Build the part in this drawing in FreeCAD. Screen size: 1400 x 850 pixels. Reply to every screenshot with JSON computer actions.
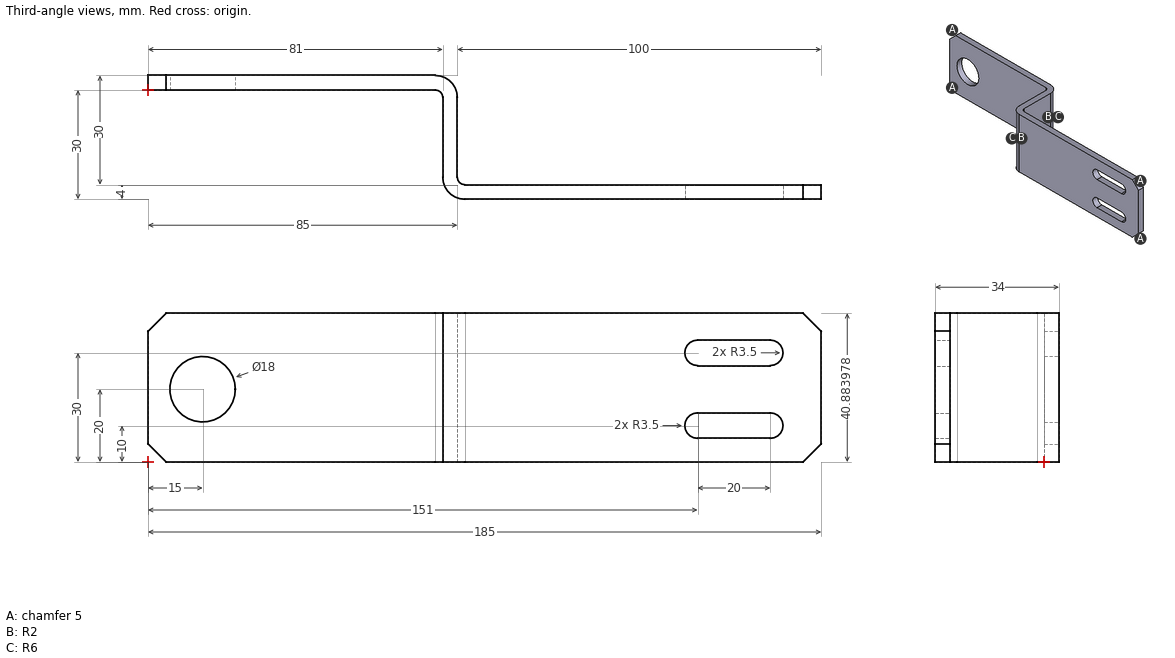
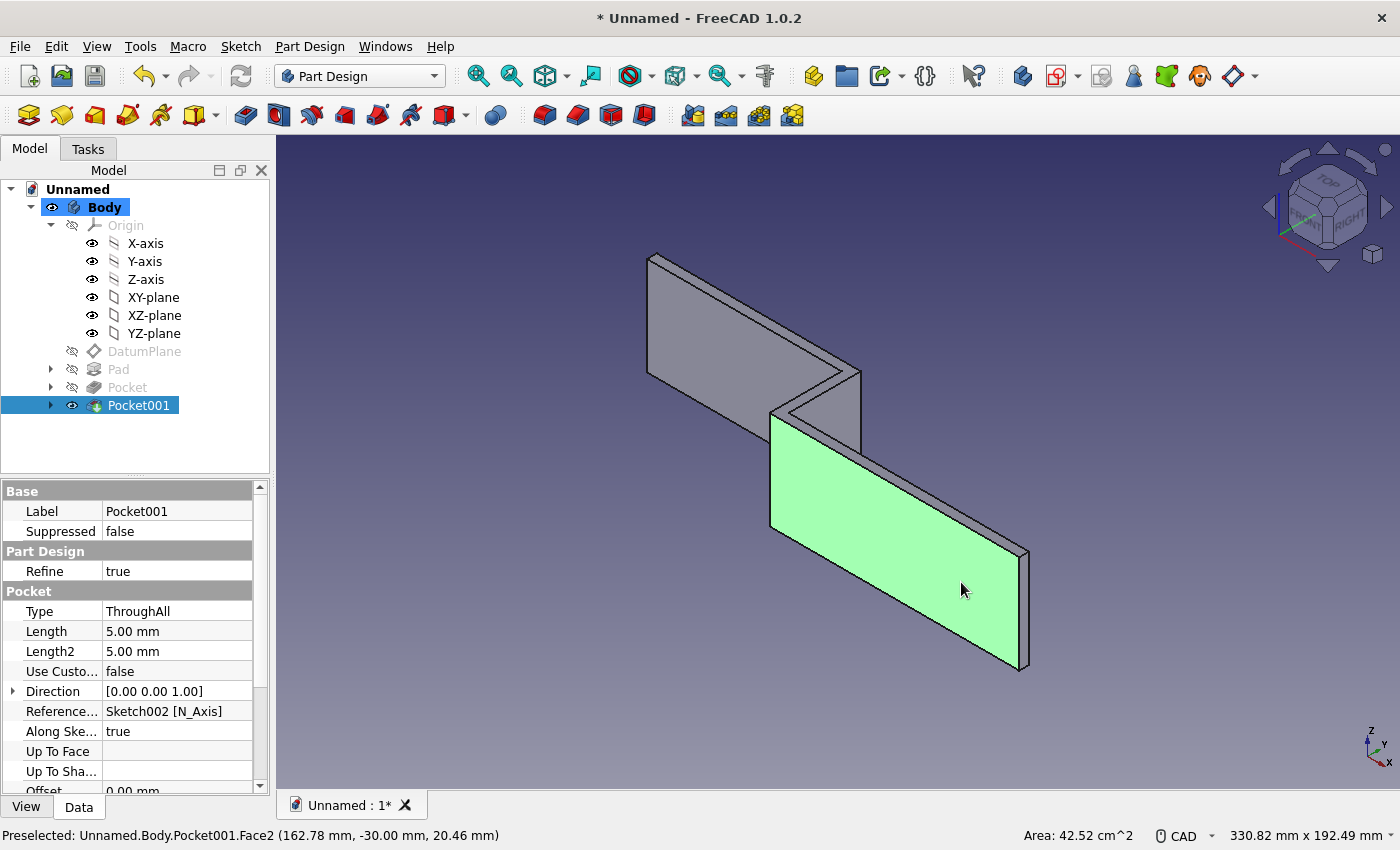
{"action": "left_click", "coordinate": [1056, 76]}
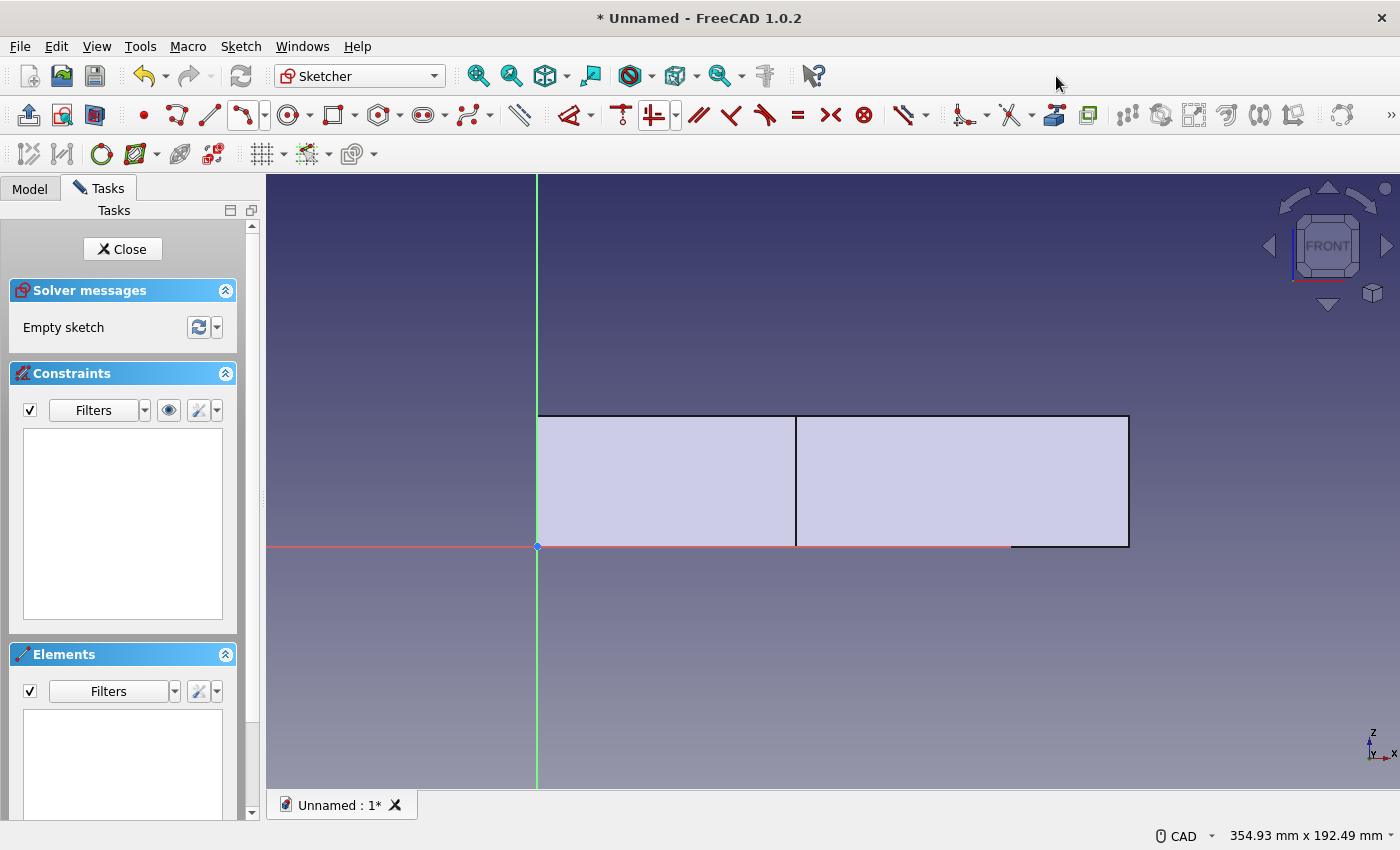
{"action": "scroll", "coordinate": [1097, 520], "scroll_direction": "up", "scroll_amount": 10}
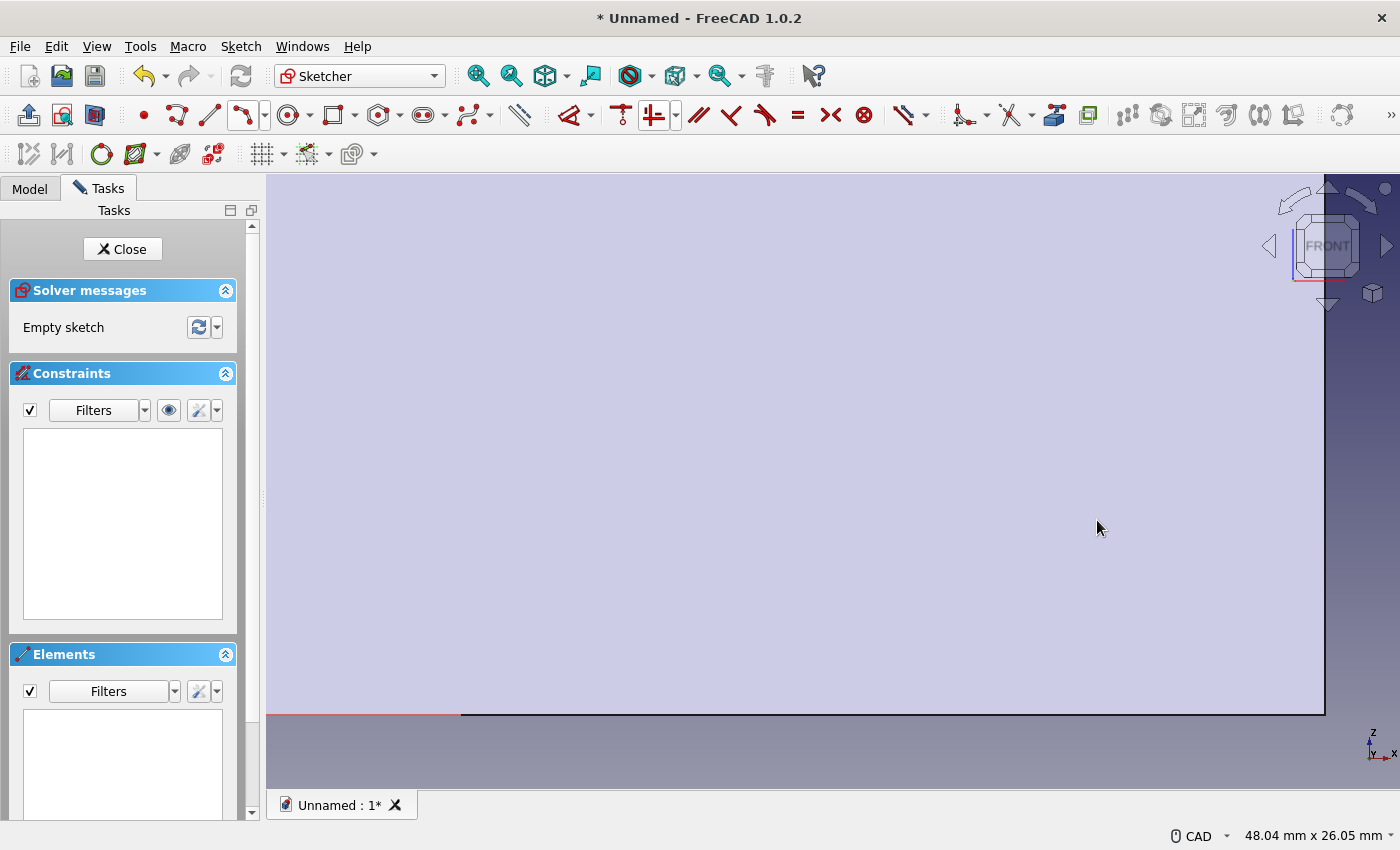
{"action": "left_click", "coordinate": [422, 116]}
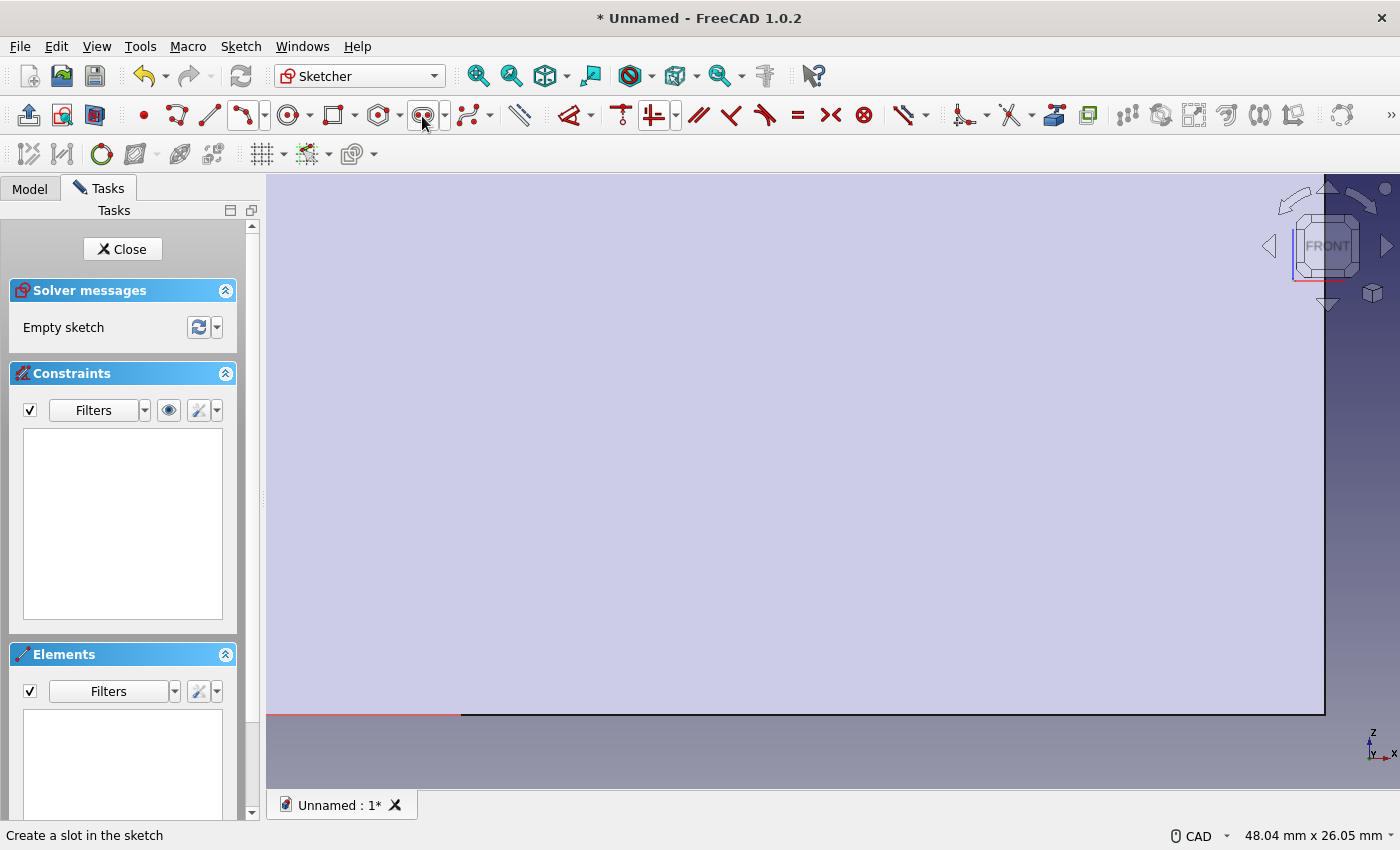
{"action": "left_click", "coordinate": [523, 478]}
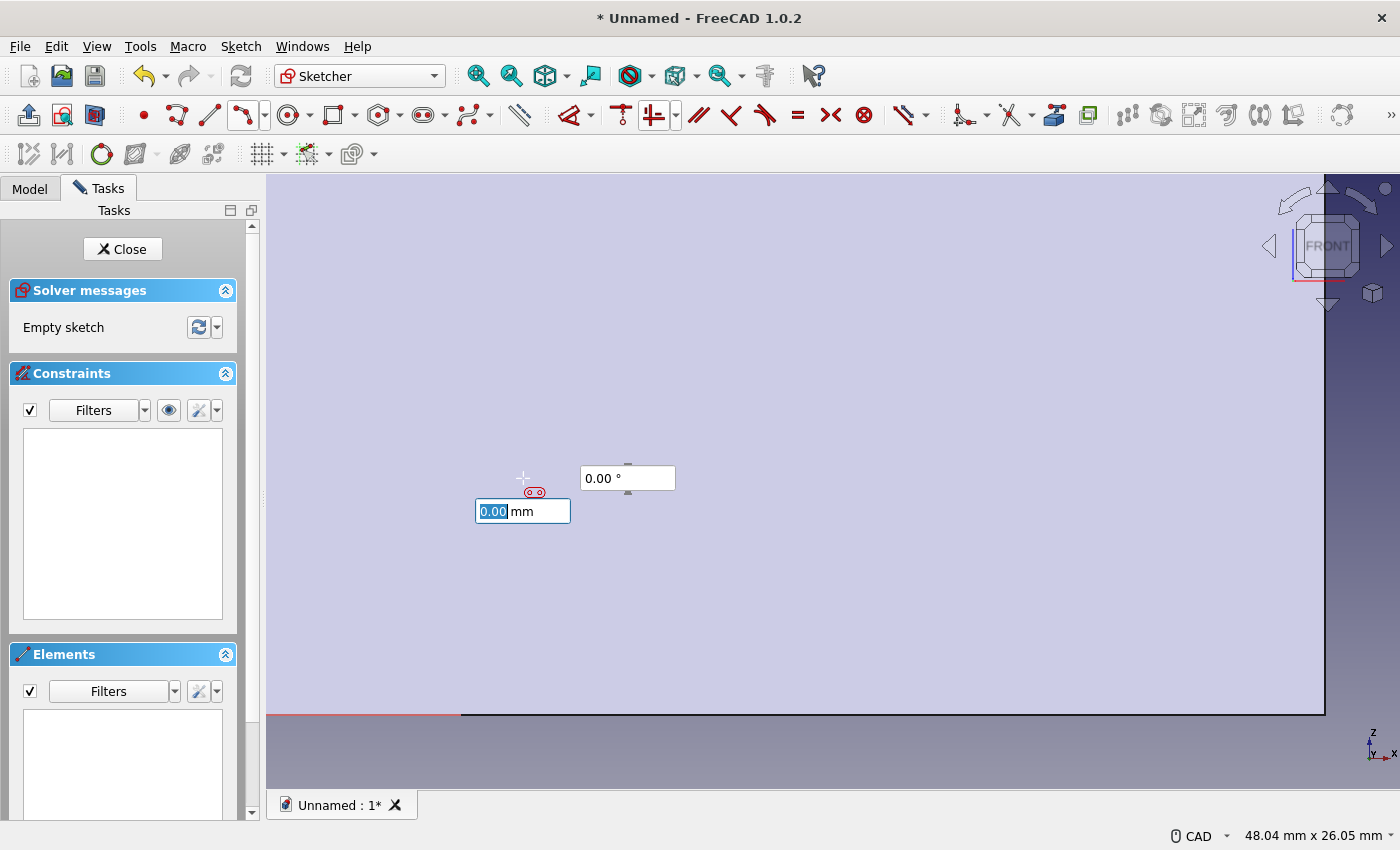
{"action": "left_click", "coordinate": [995, 478]}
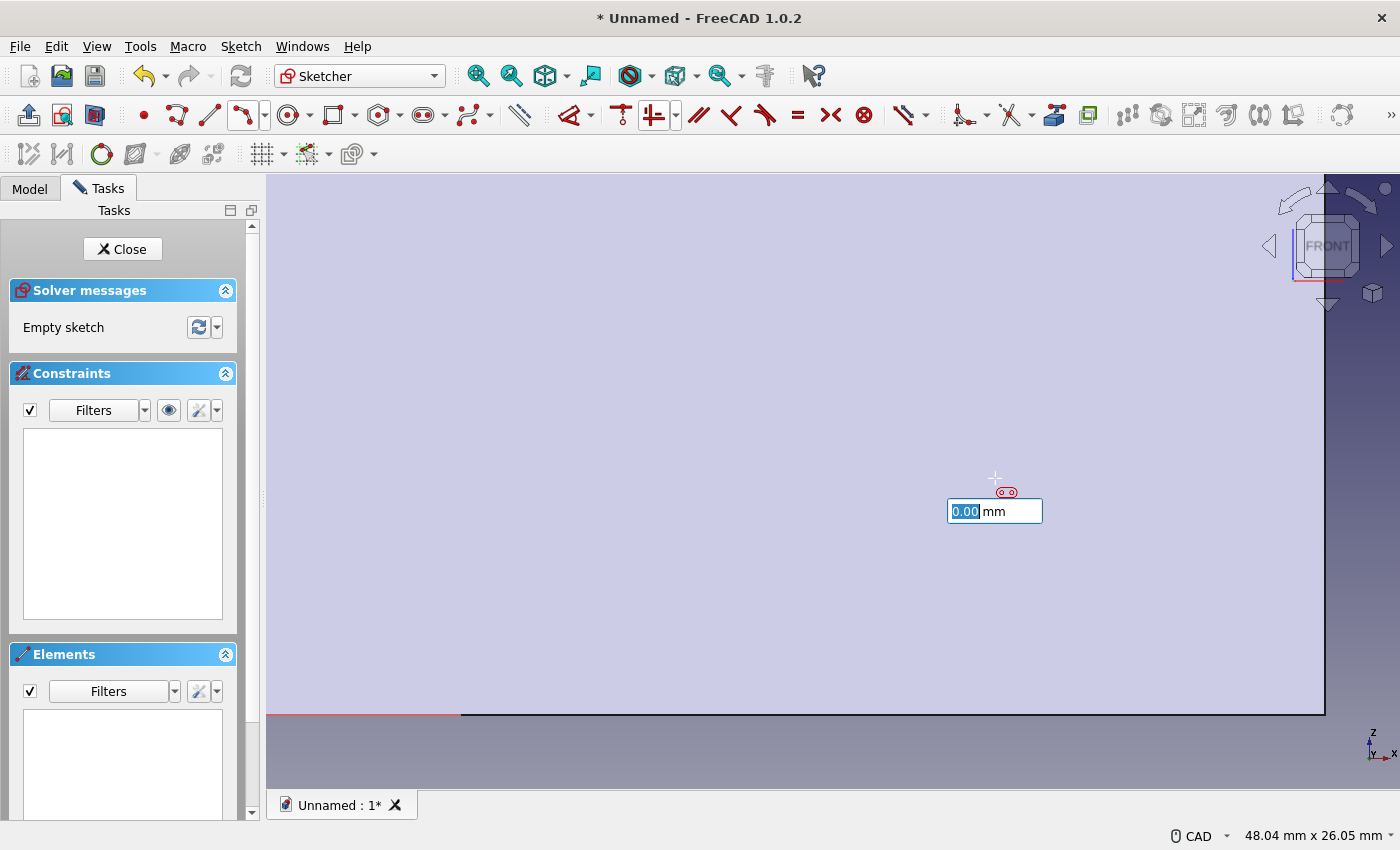
{"action": "left_click", "coordinate": [759, 396]}
{"action": "key", "text": "Escape"}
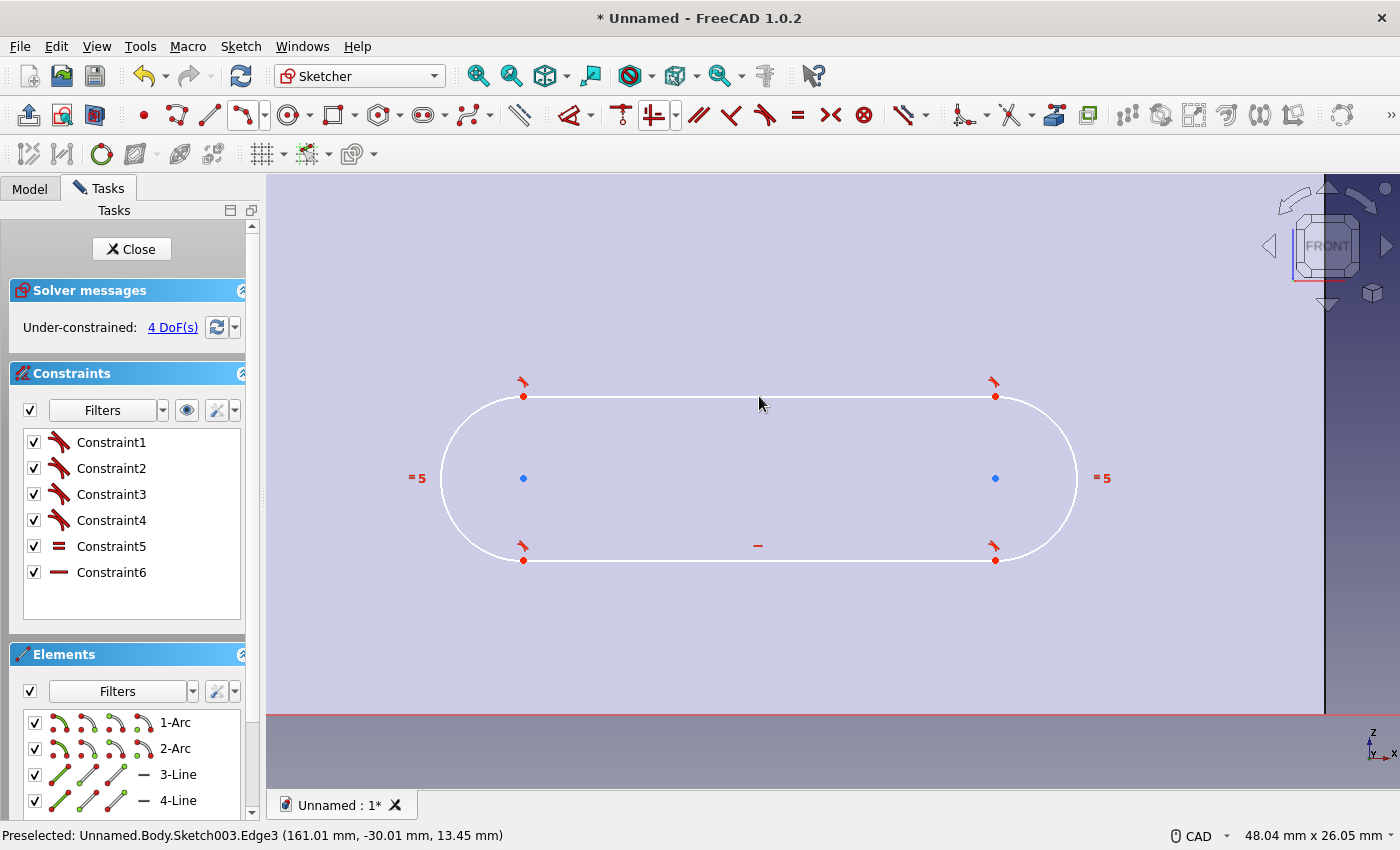
{"action": "left_click", "coordinate": [568, 116]}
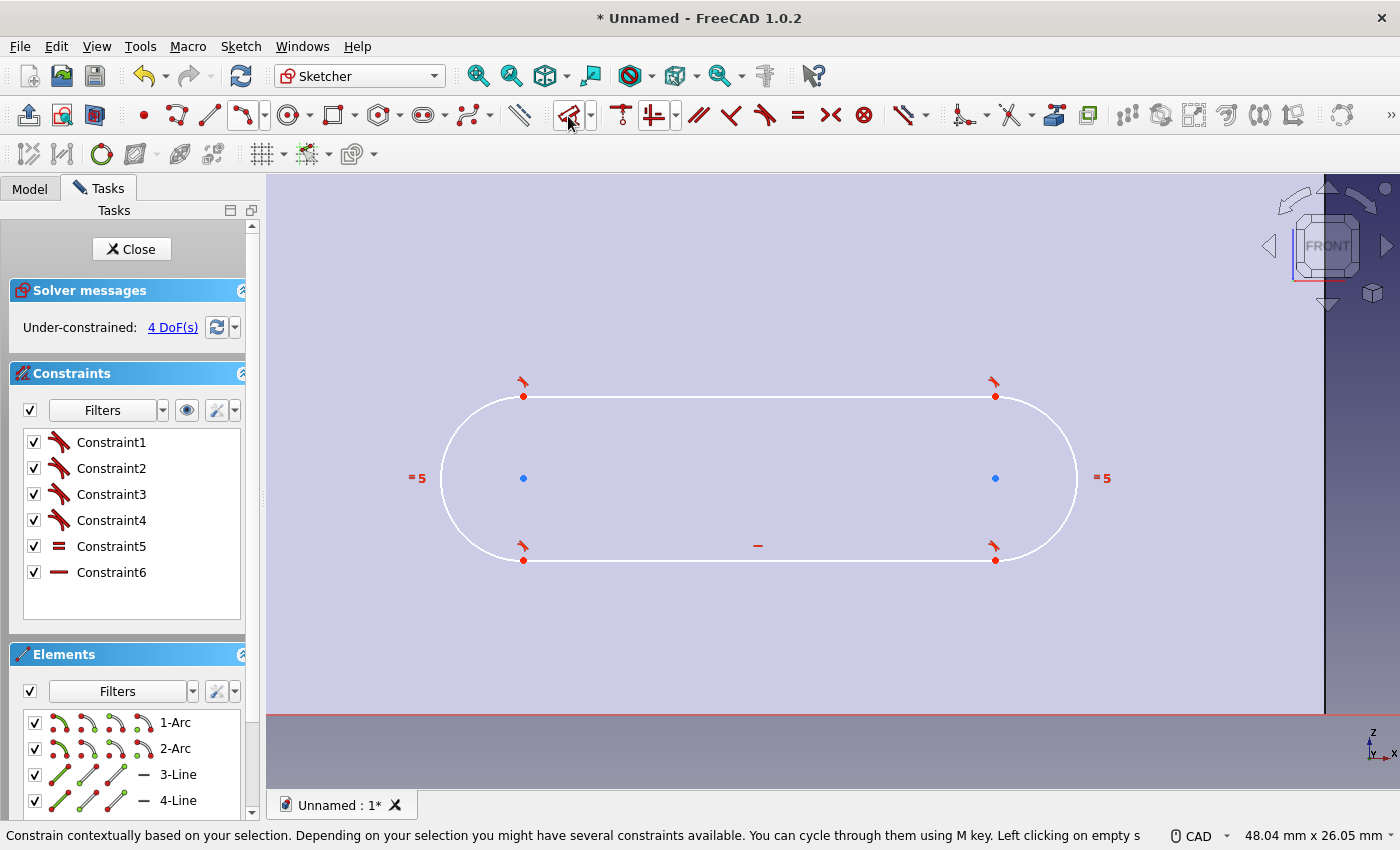
{"action": "left_click", "coordinate": [457, 431]}
{"action": "left_click", "coordinate": [431, 412]}